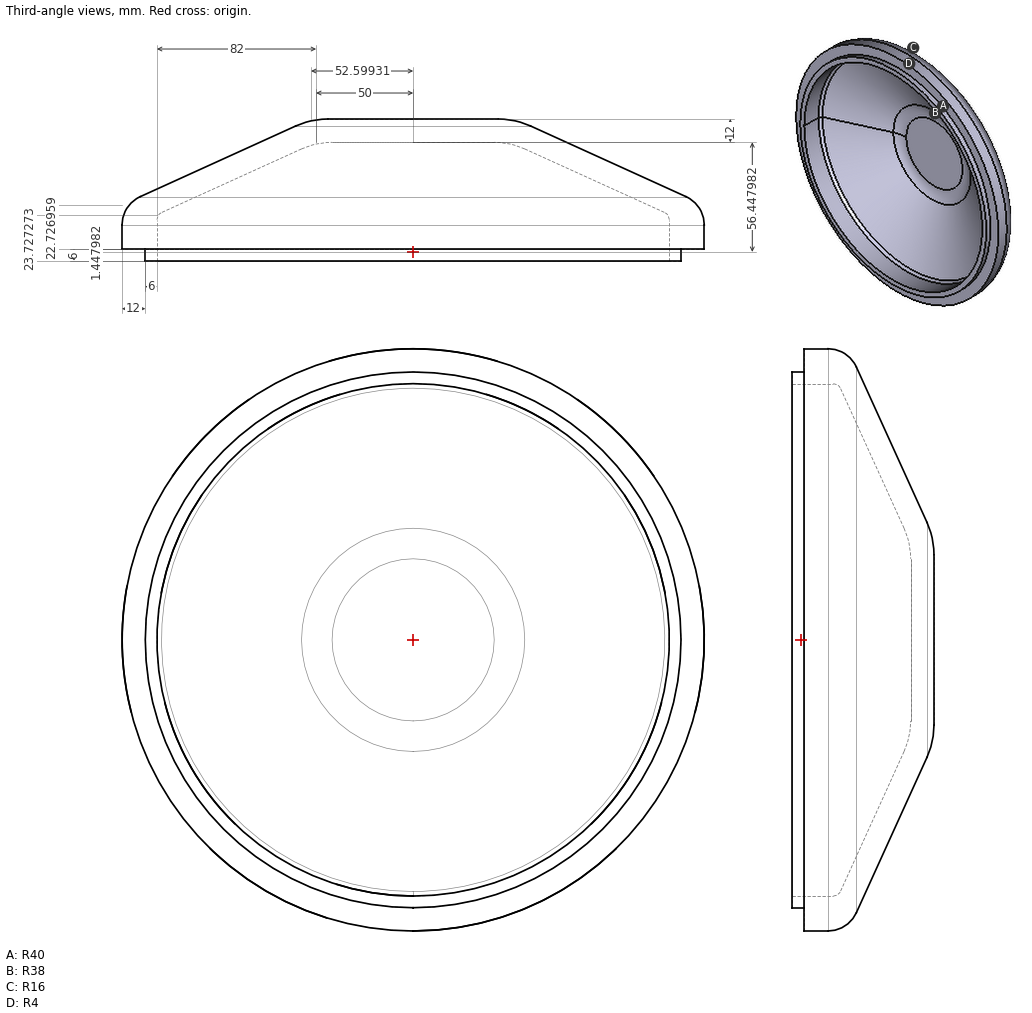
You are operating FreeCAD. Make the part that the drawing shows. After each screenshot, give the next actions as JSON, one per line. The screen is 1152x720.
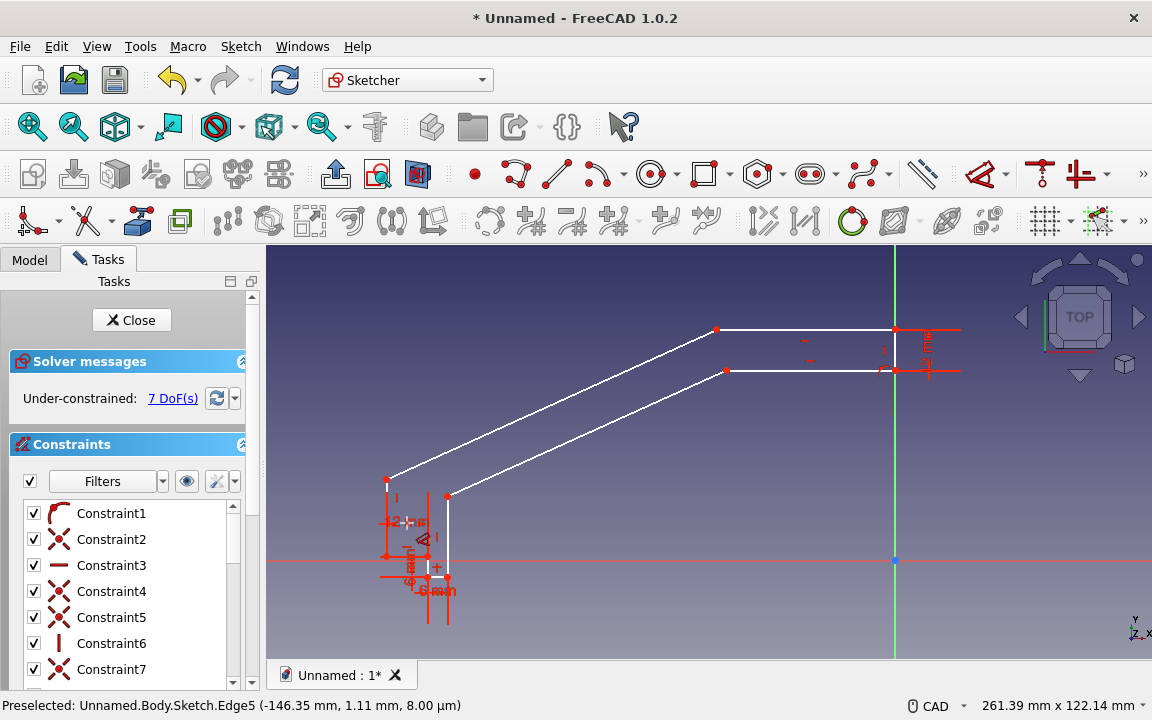
{"action": "left_click", "coordinate": [777, 371]}
{"action": "left_click", "coordinate": [811, 405]}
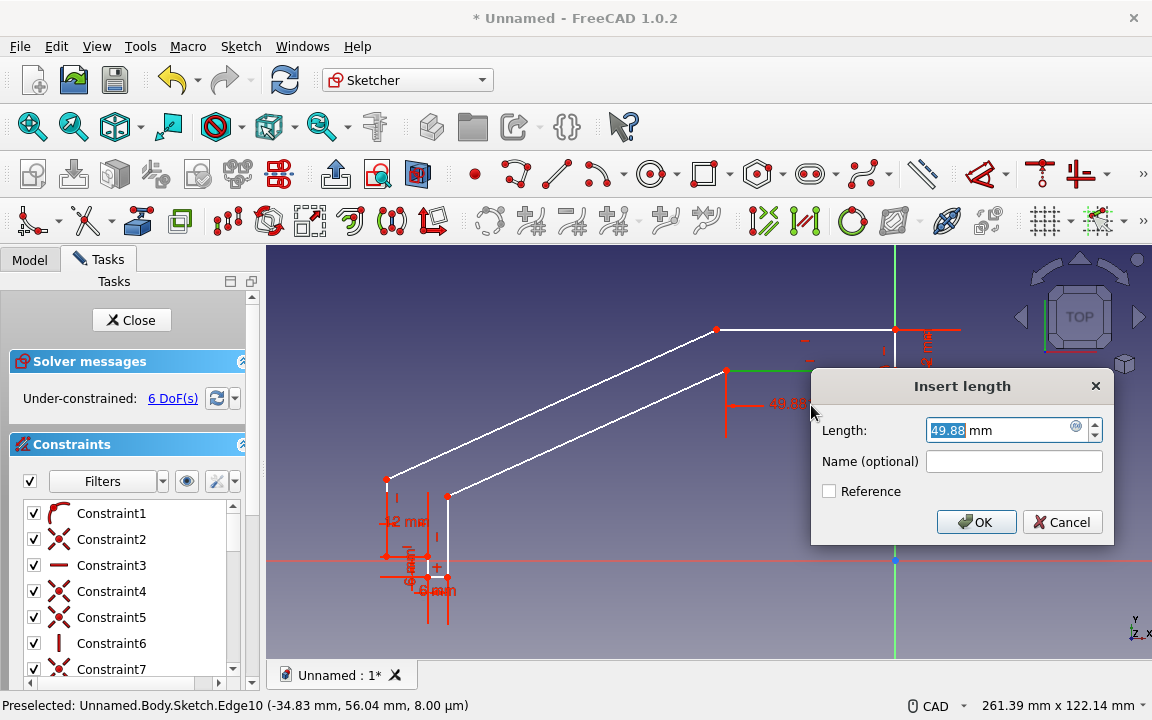
{"action": "type", "text": "50"}
{"action": "key", "text": "Return"}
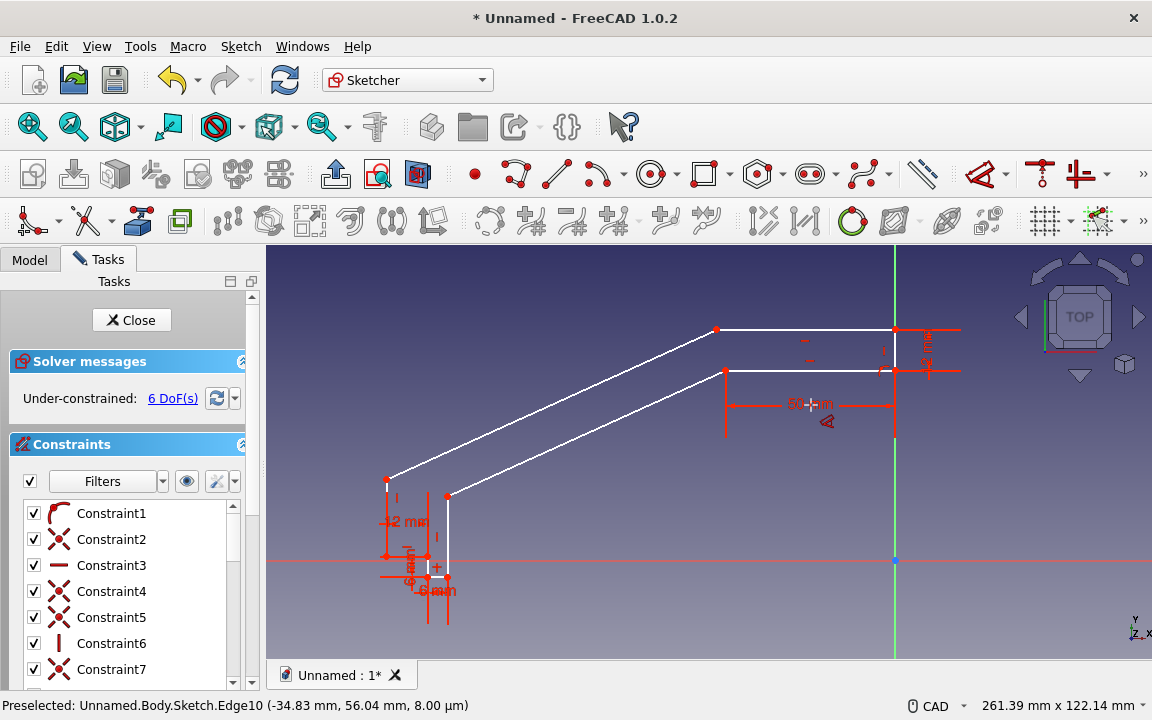
{"action": "left_click", "coordinate": [531, 459]}
{"action": "left_click", "coordinate": [587, 337]}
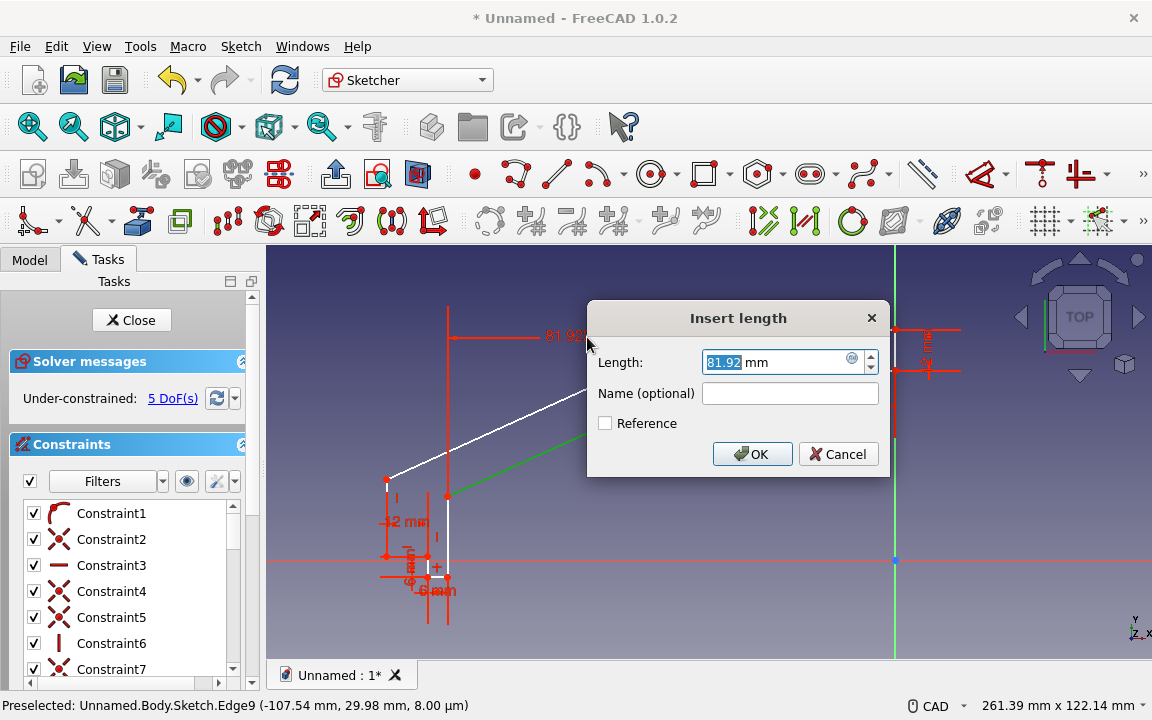
{"action": "type", "text": "82"}
{"action": "key", "text": "Return"}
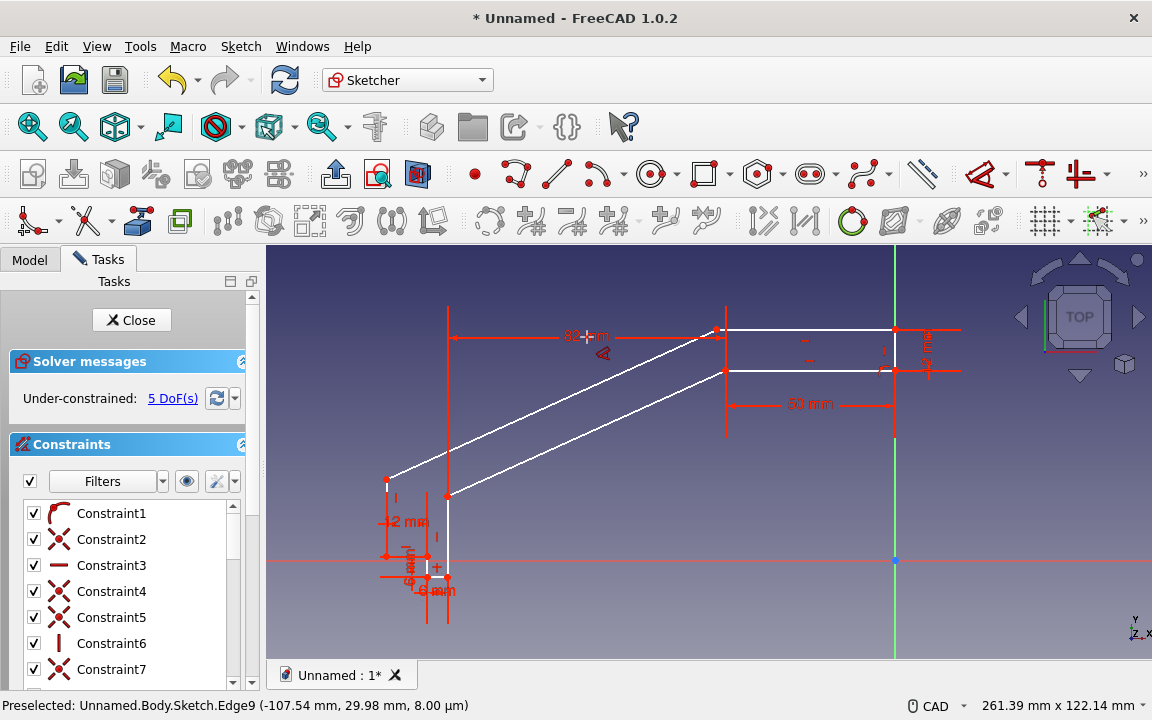
{"action": "left_click", "coordinate": [842, 330]}
{"action": "left_click", "coordinate": [806, 296]}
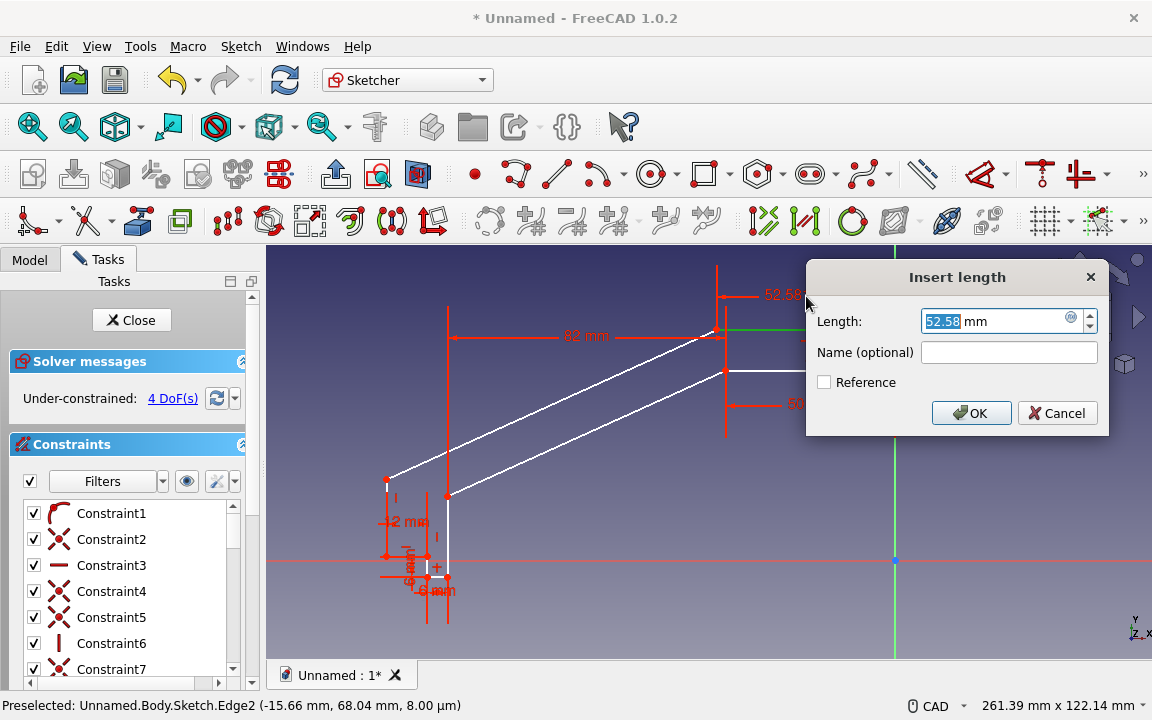
{"action": "type", "text": "52.59931"}
{"action": "key", "text": "Return"}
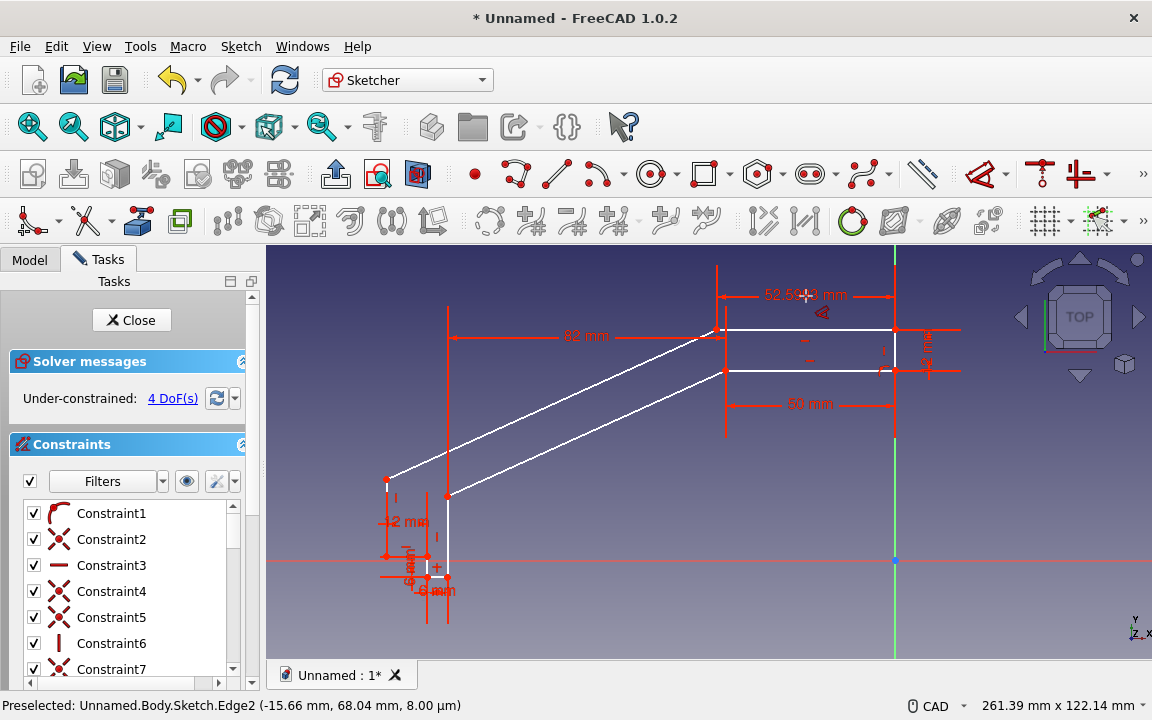
{"action": "left_click", "coordinate": [387, 503]}
{"action": "left_click", "coordinate": [353, 500]}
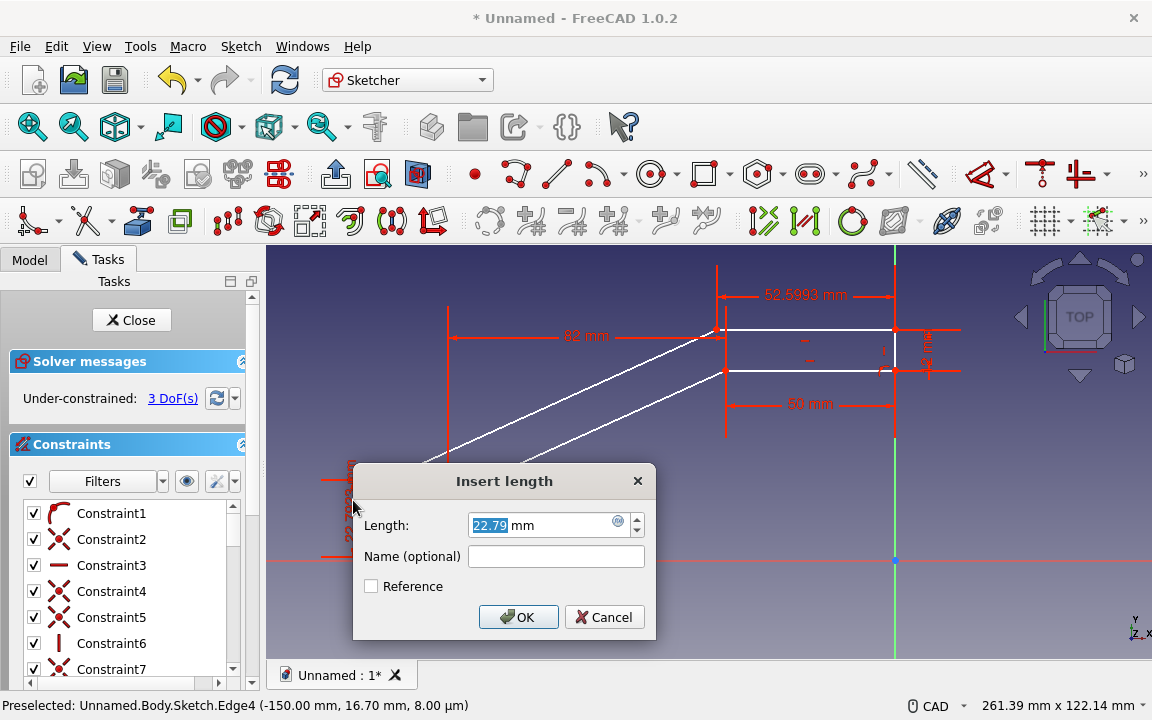
{"action": "type", "text": "22.726959"}
{"action": "key", "text": "Return"}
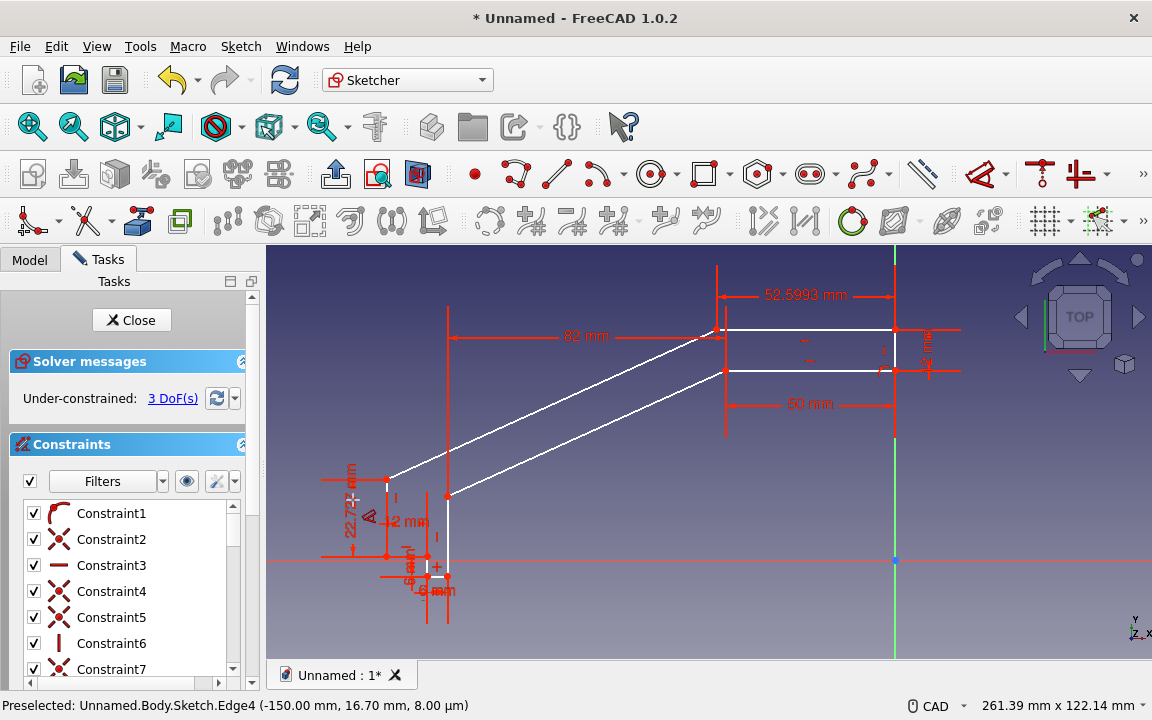
{"action": "left_click", "coordinate": [448, 521]}
{"action": "left_click", "coordinate": [482, 537]}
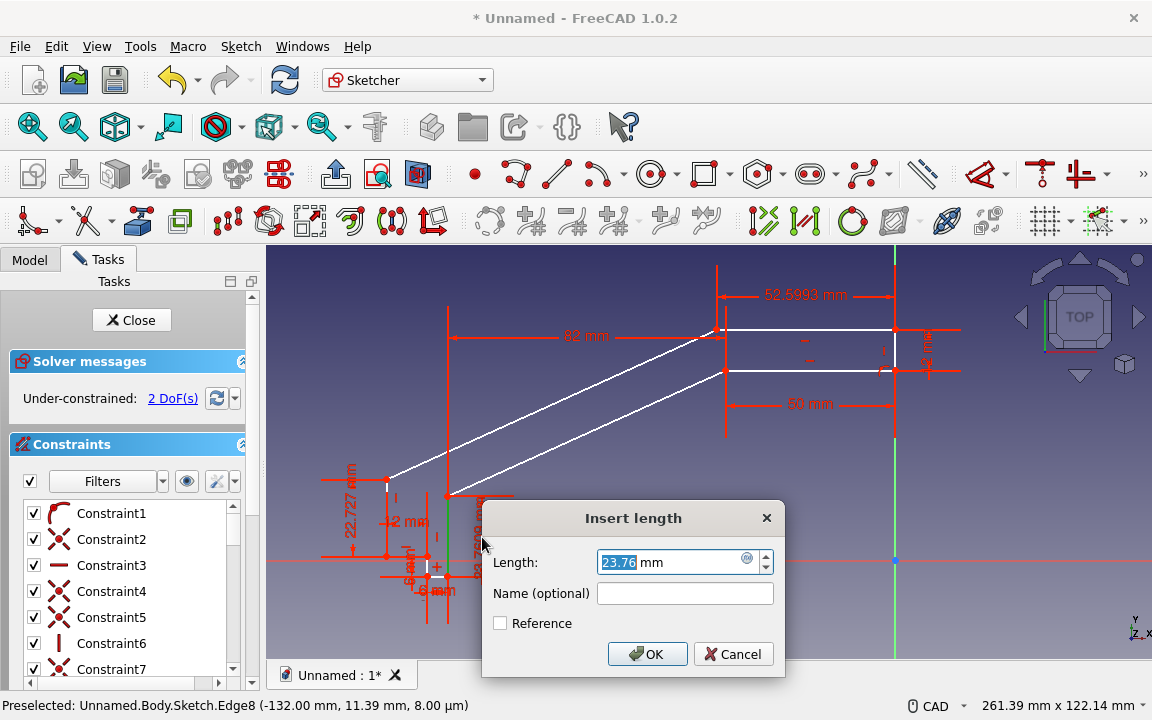
{"action": "type", "text": "23.727273"}
{"action": "key", "text": "Return"}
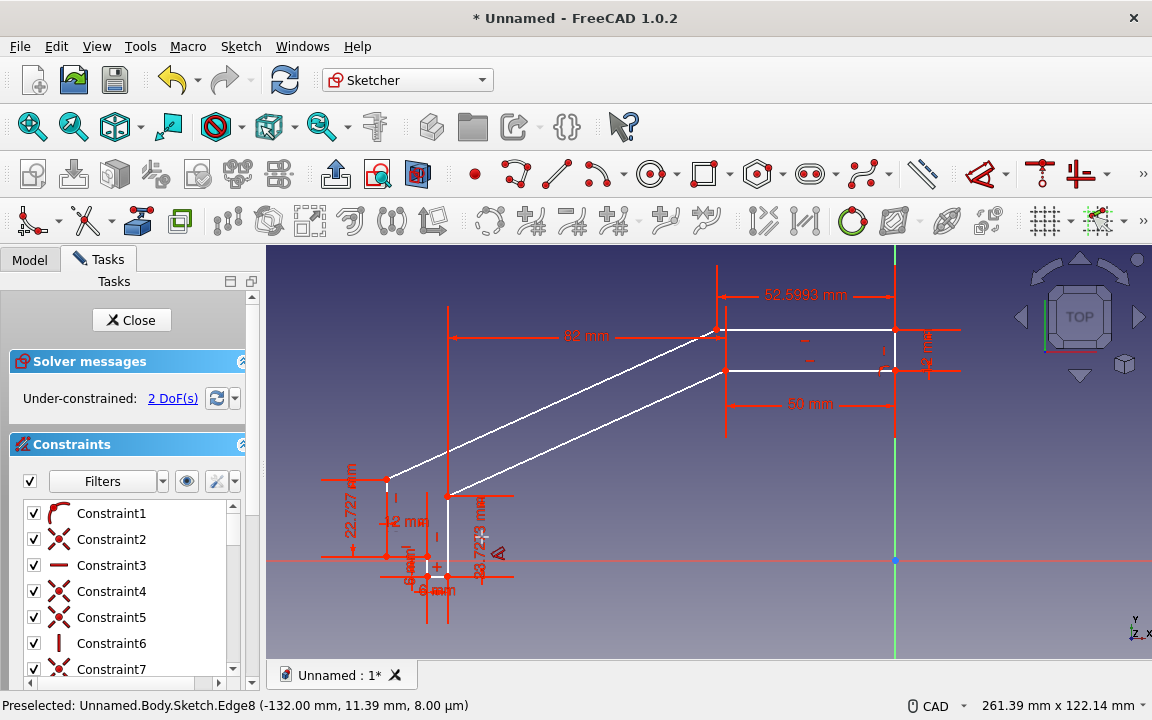
{"action": "scroll", "coordinate": [387, 557], "scroll_direction": "up", "scroll_amount": 11}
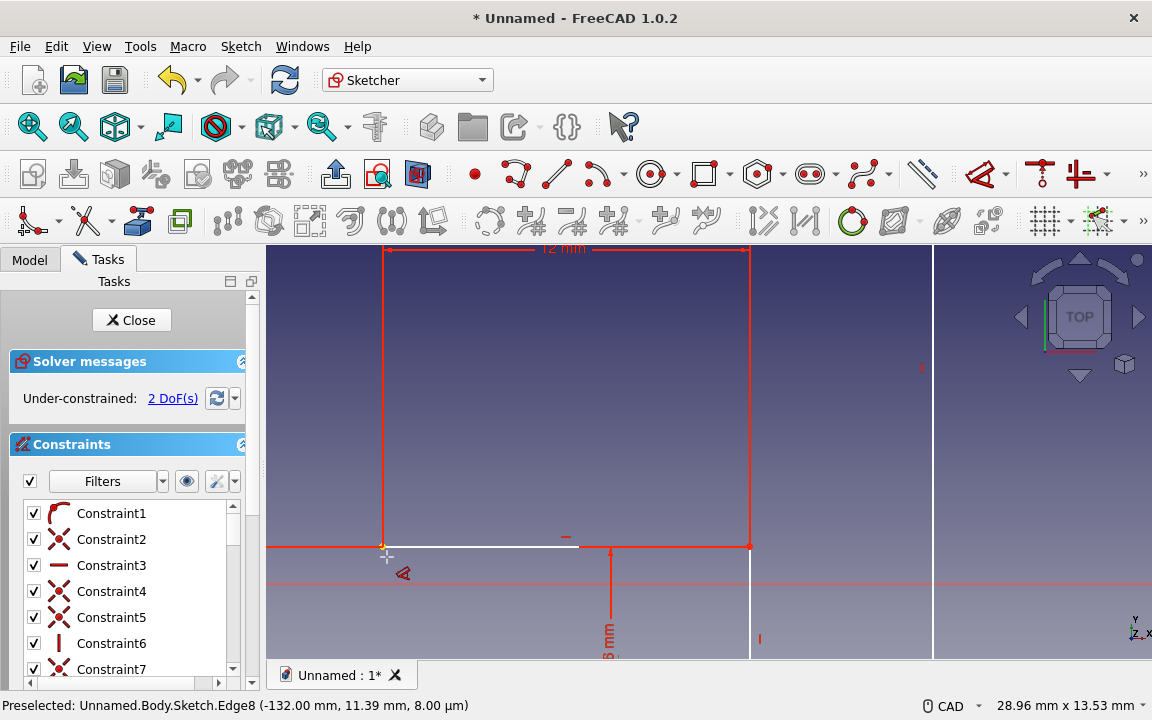
{"action": "left_click", "coordinate": [383, 547]}
{"action": "left_click", "coordinate": [349, 565]}